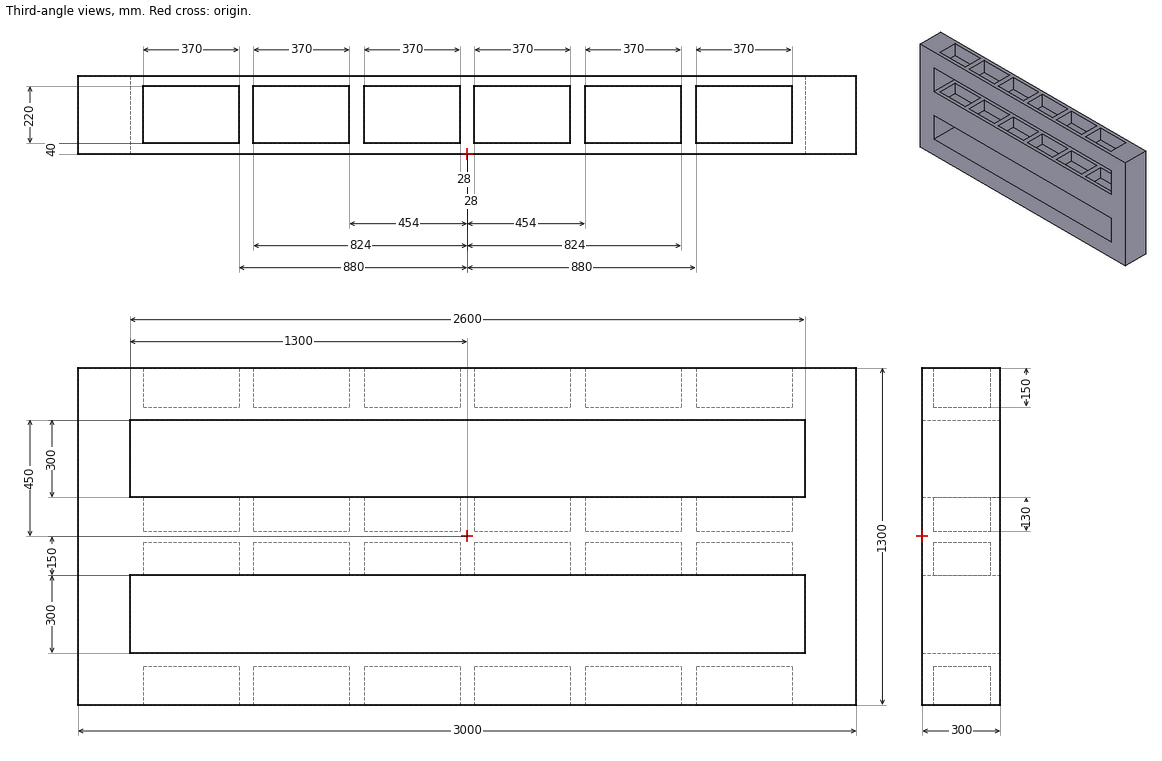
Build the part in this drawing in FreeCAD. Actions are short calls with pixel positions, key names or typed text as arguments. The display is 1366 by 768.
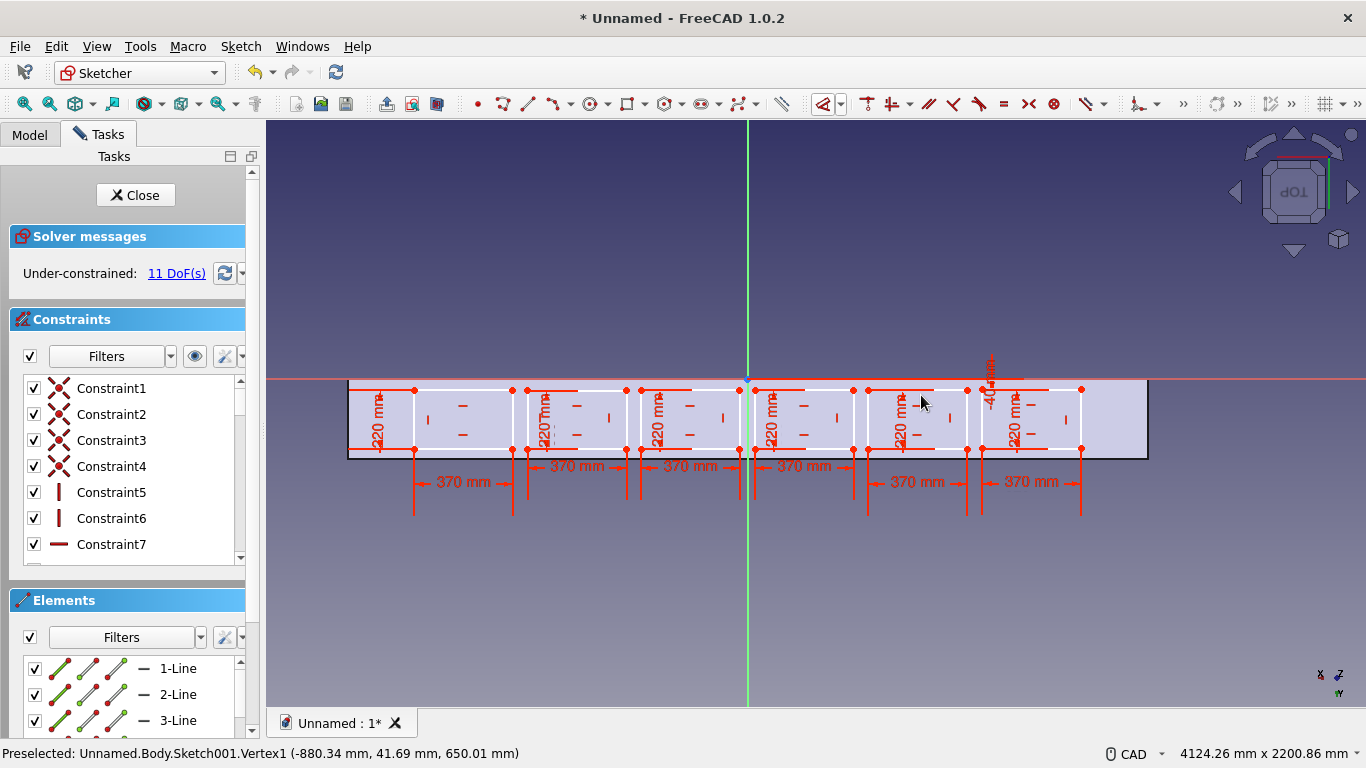
scroll(414, 390, up, 7)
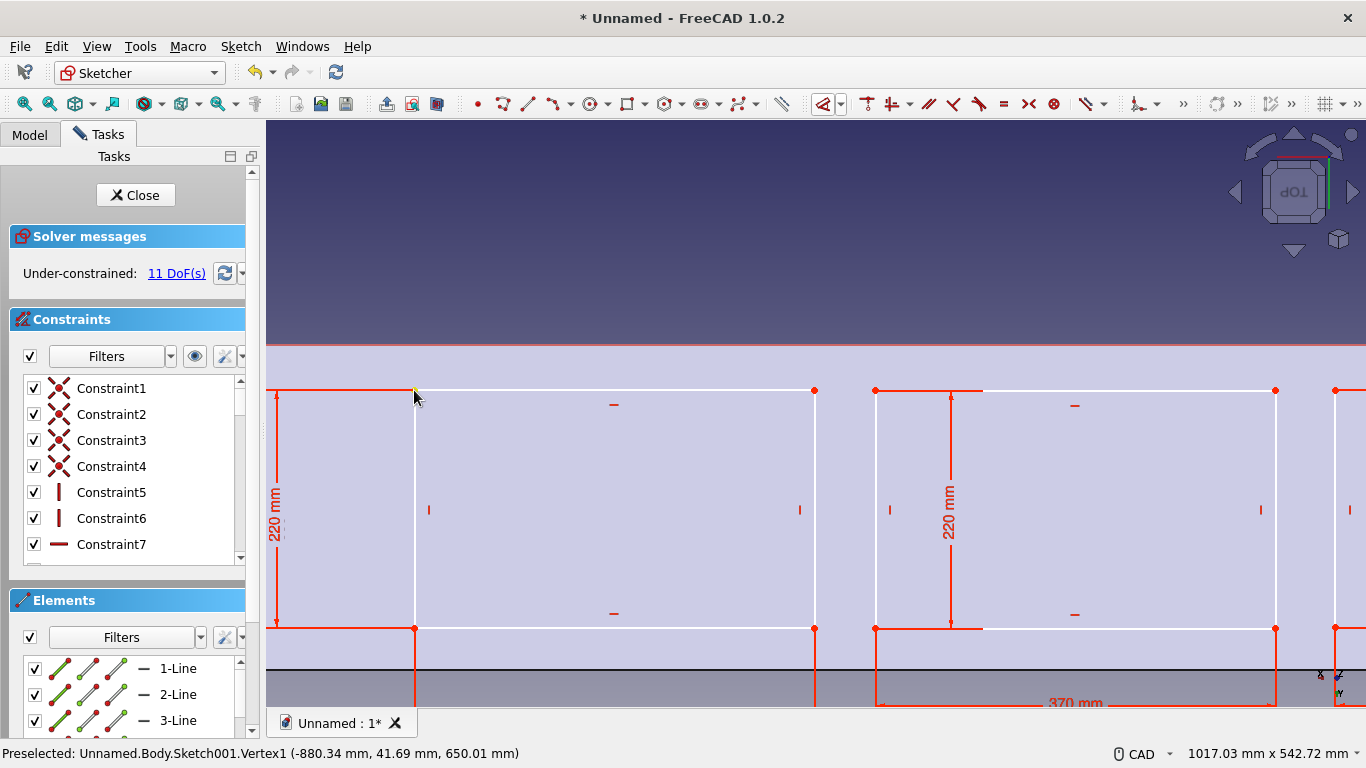
click(415, 390)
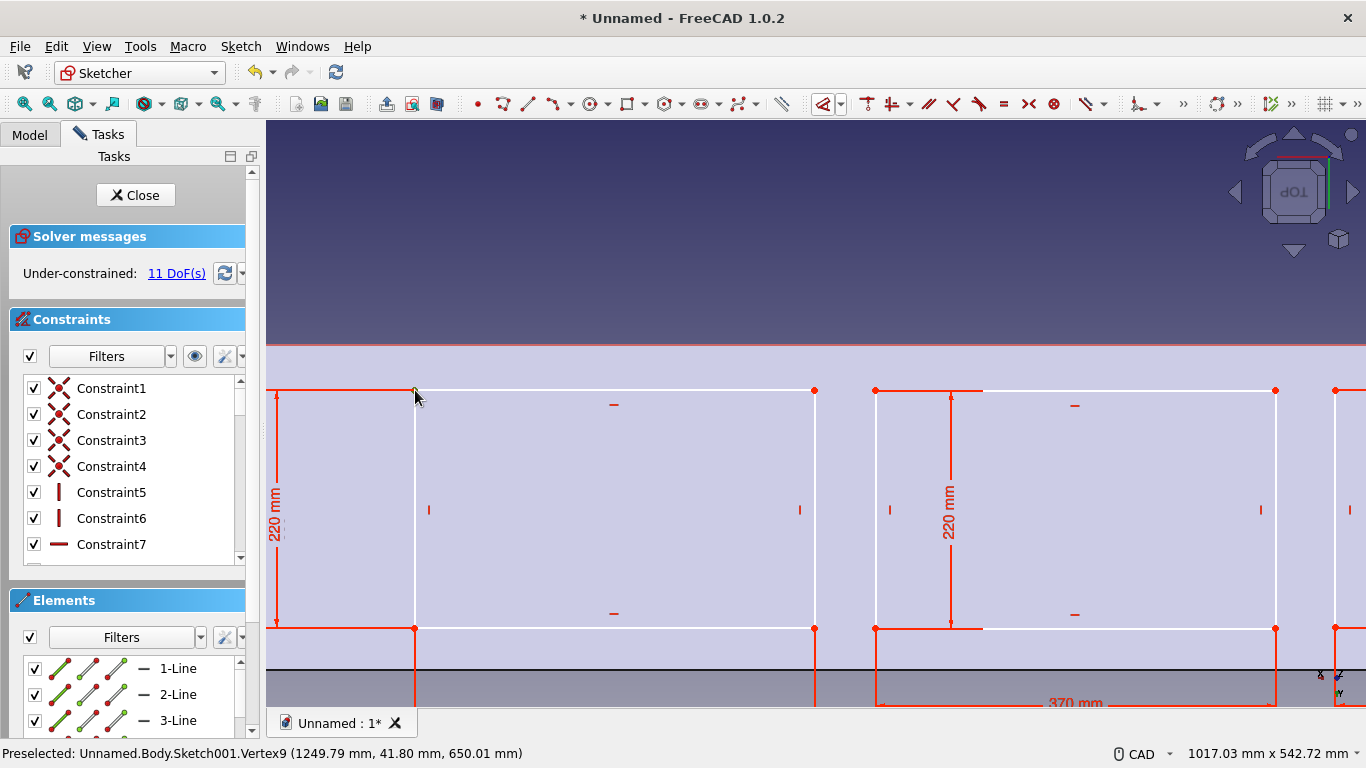
key(i)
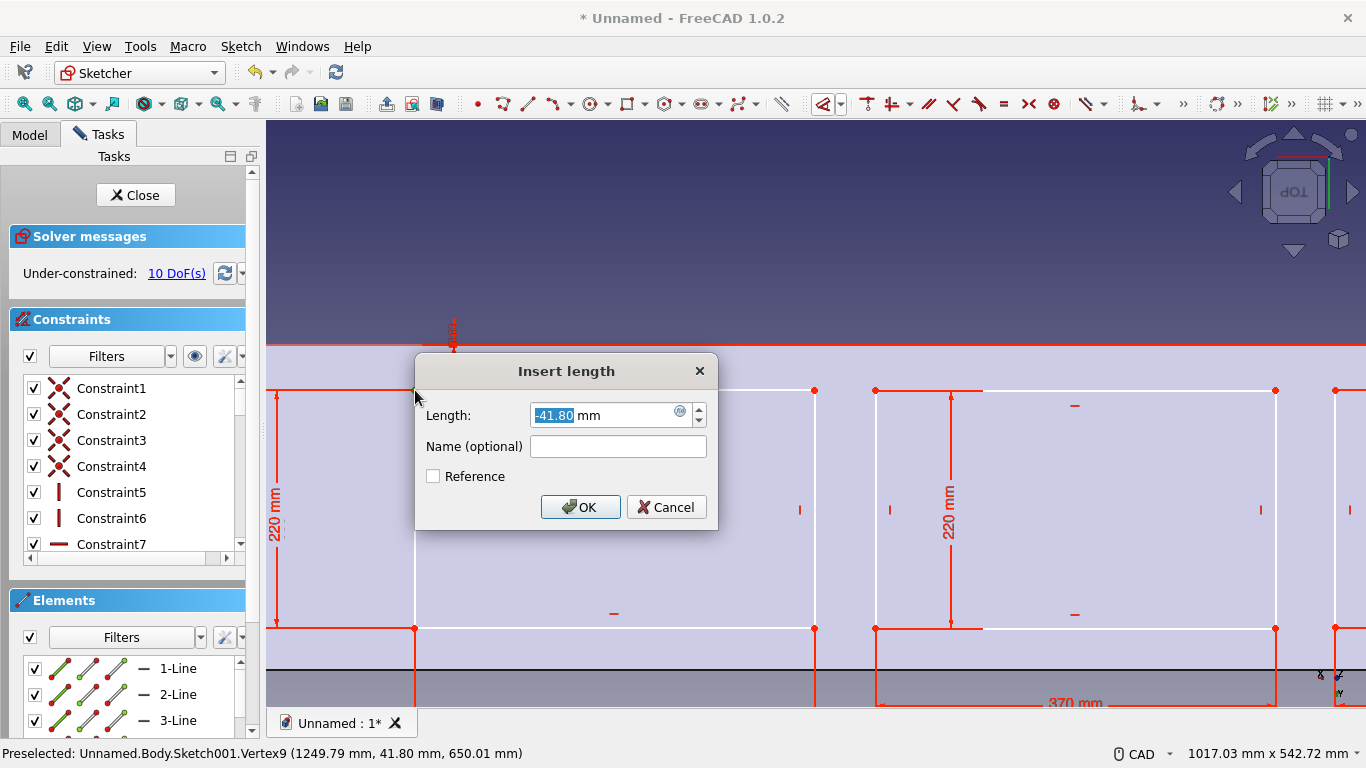
text(-40)
key(Return)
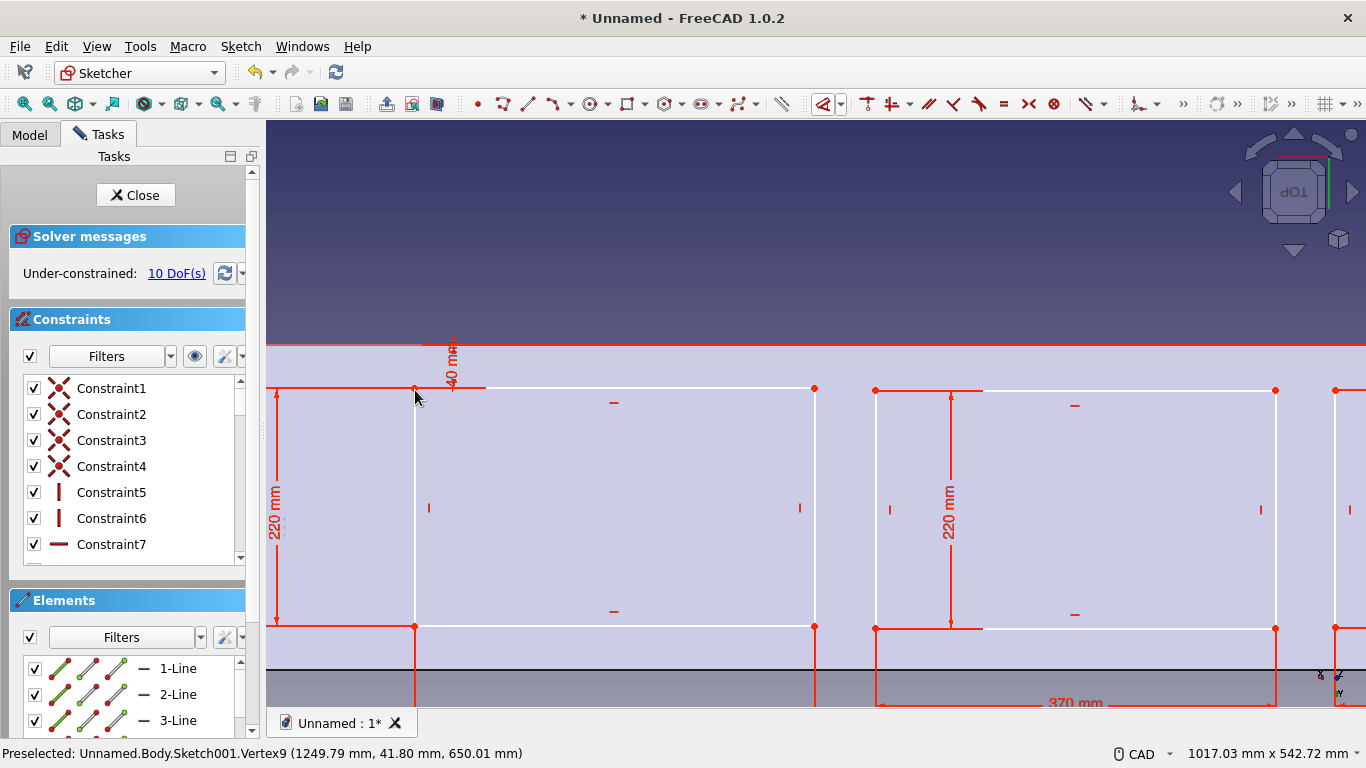
scroll(414, 390, down, 7)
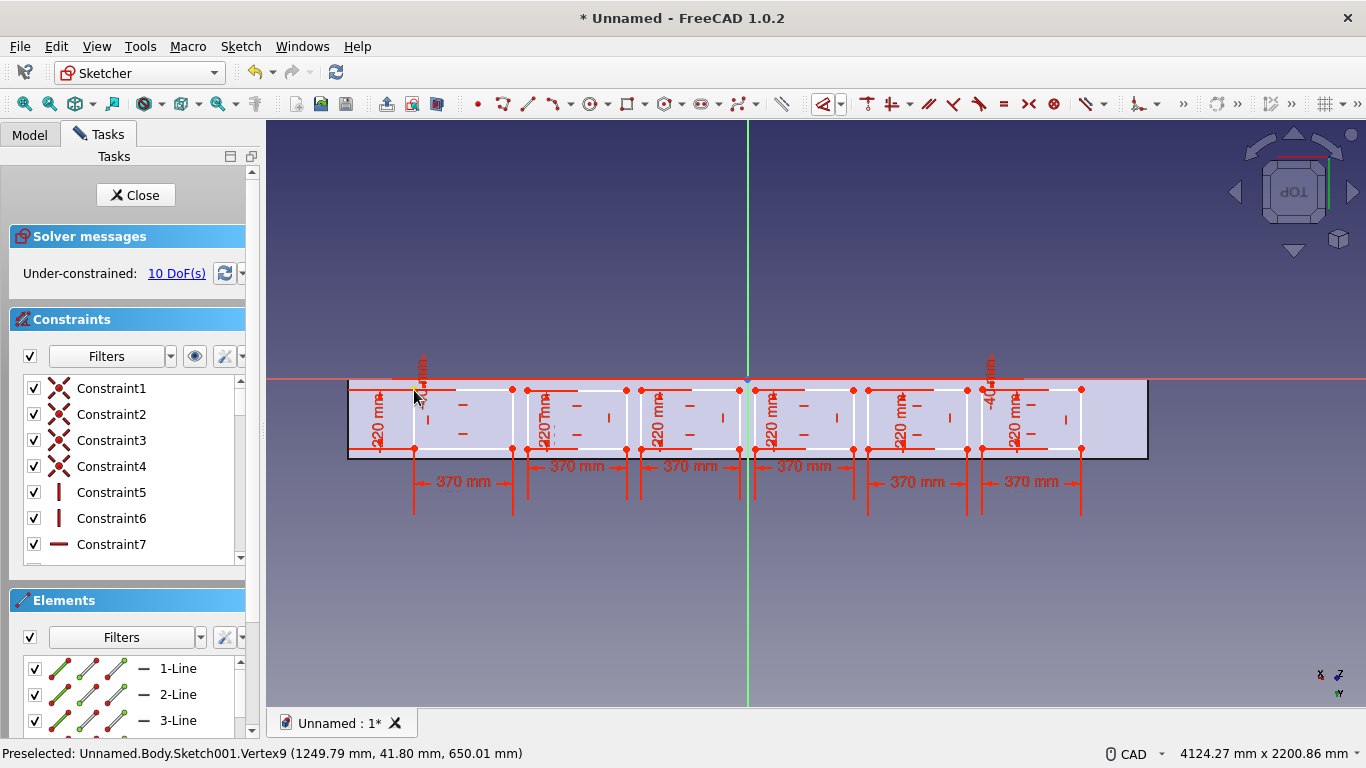
scroll(868, 390, up, 7)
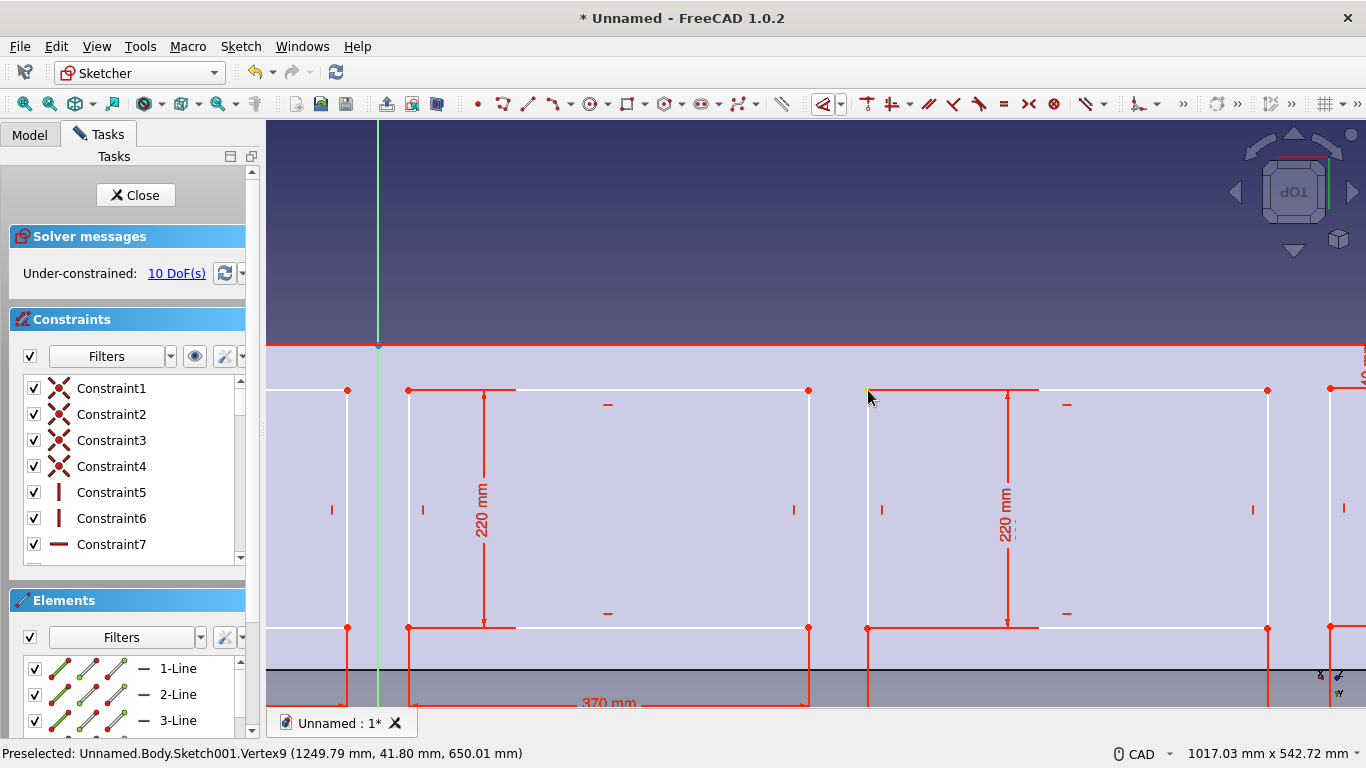
click(868, 390)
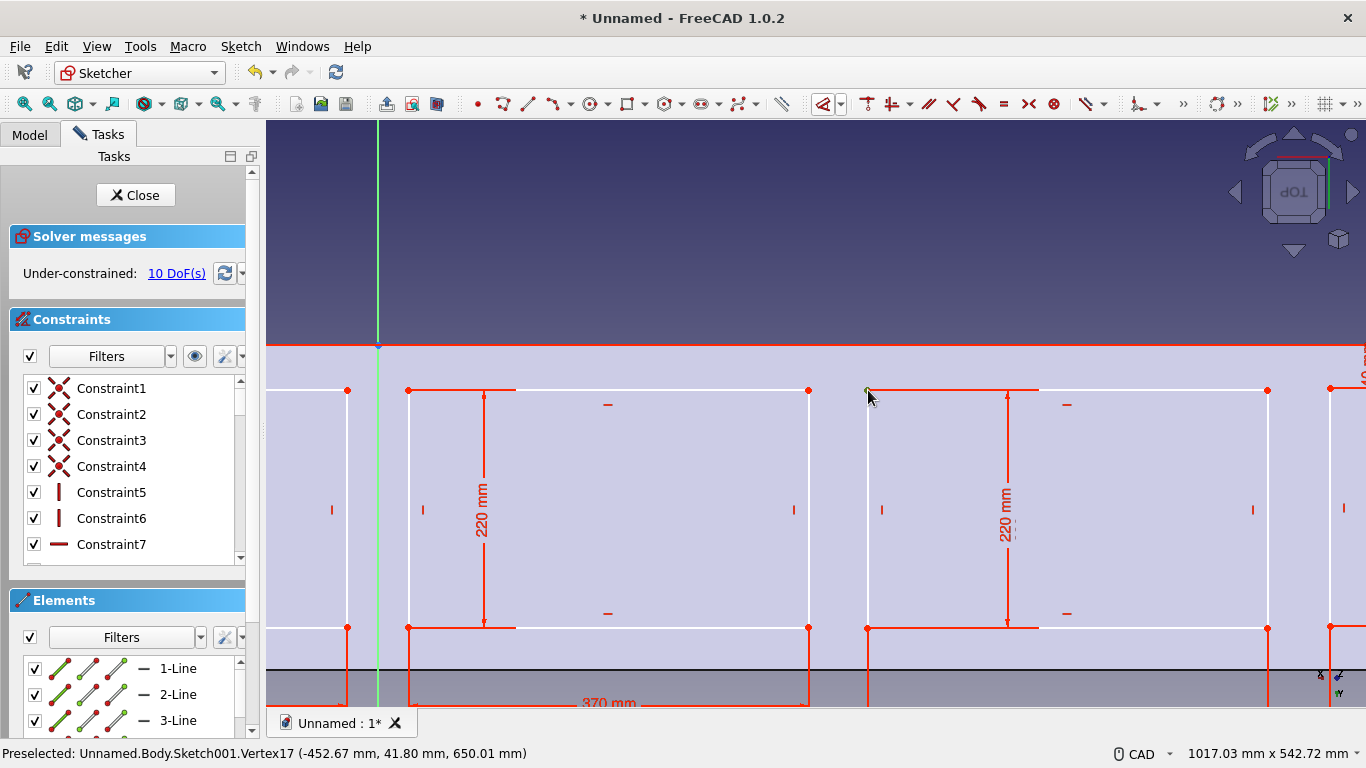
key(i)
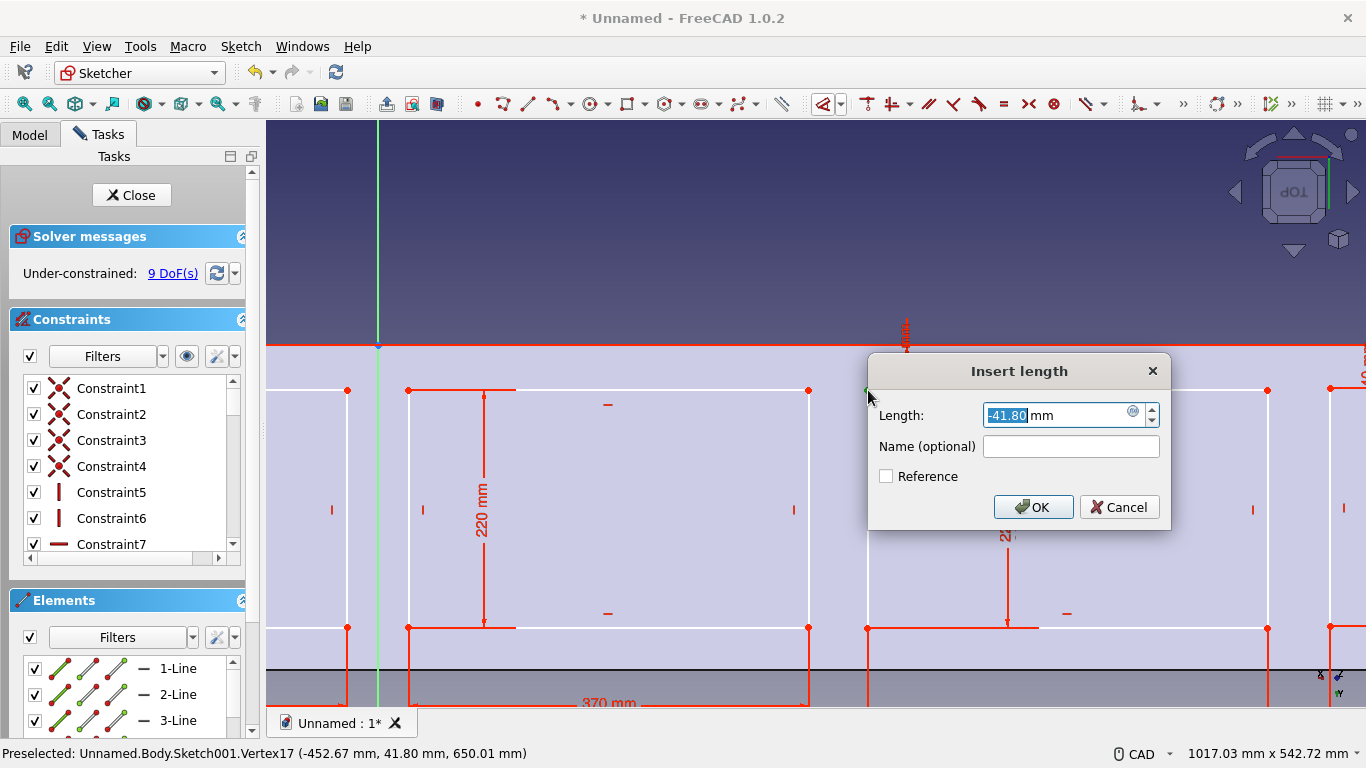
text(-40)
key(Return)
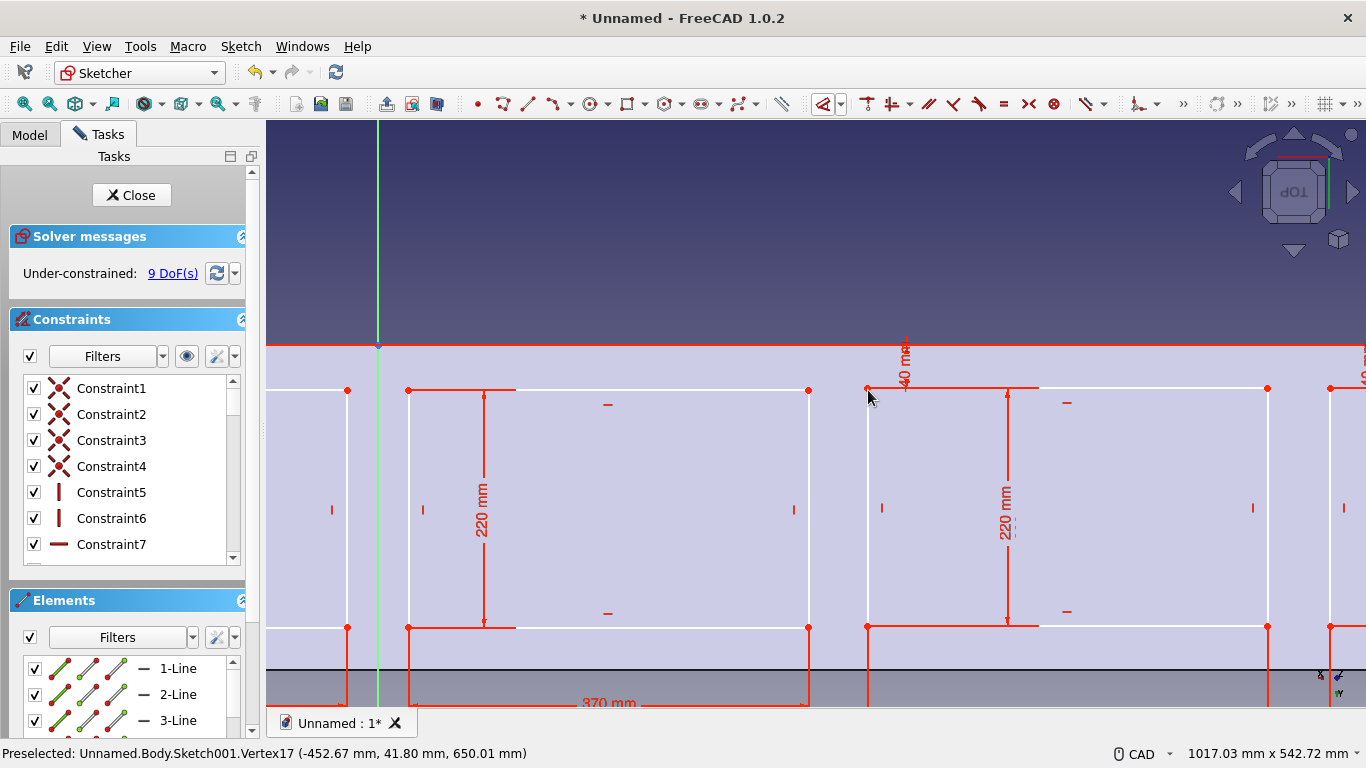
scroll(409, 390, up, 2)